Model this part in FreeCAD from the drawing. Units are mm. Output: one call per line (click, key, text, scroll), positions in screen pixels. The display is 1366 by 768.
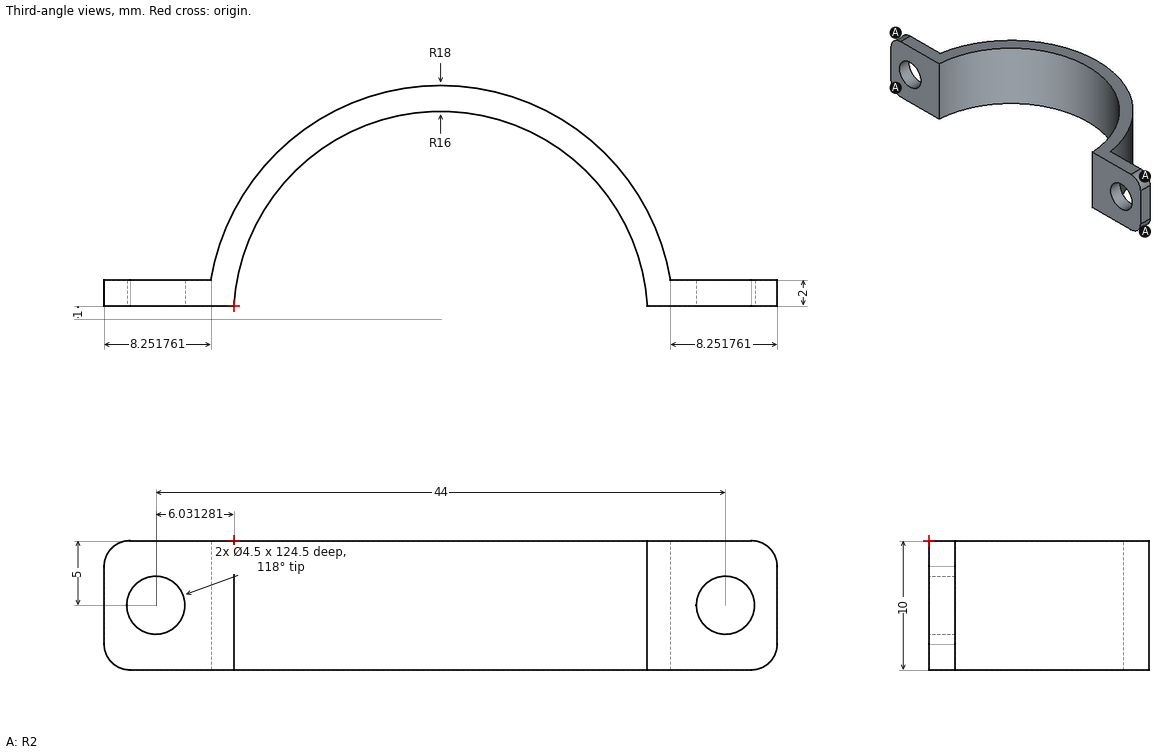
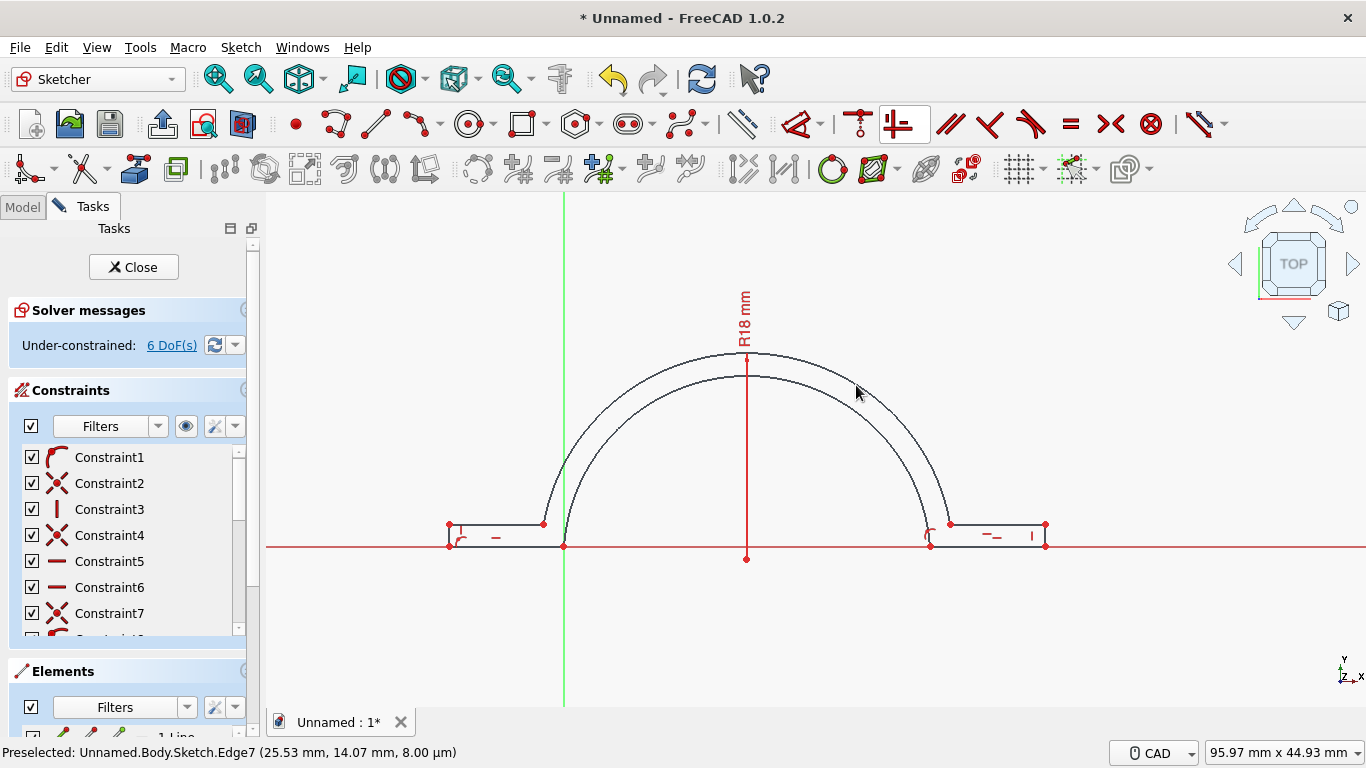
click(851, 408)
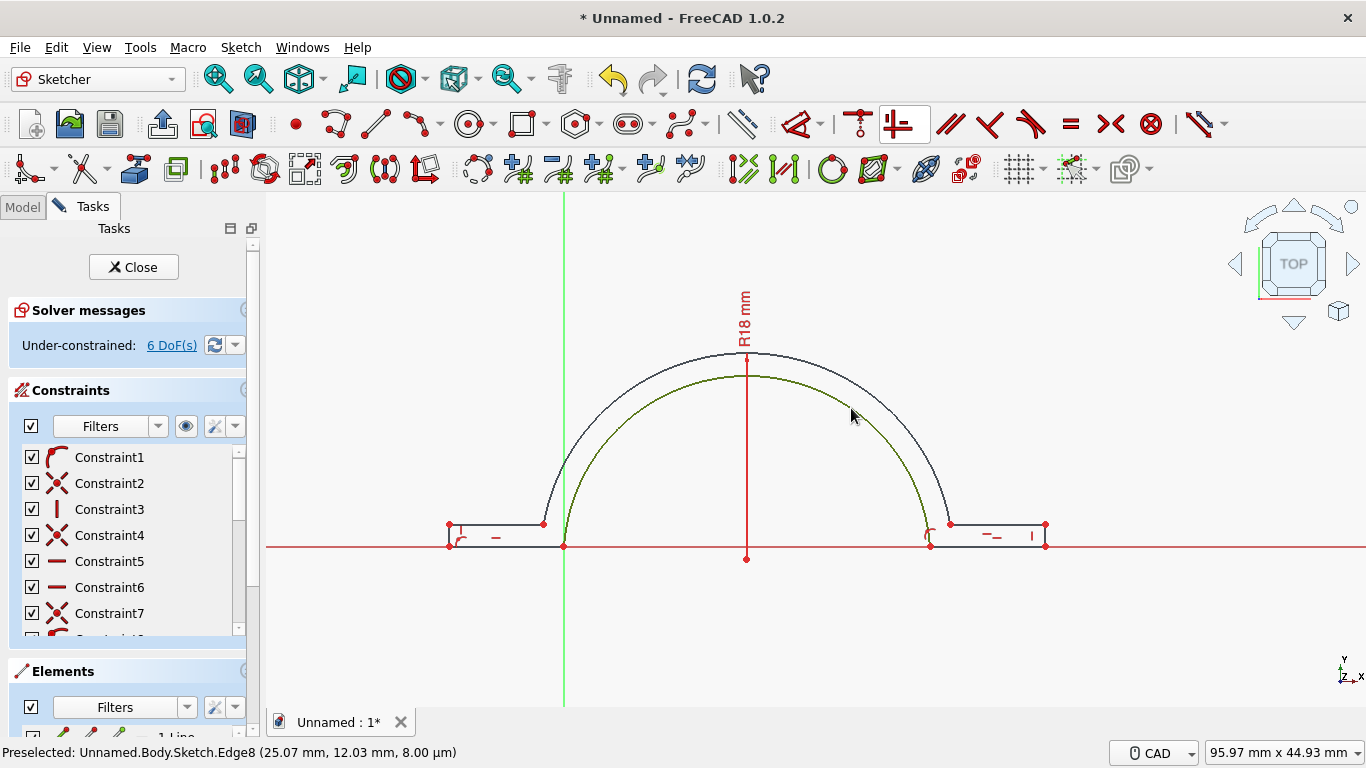
key(k)
key(r)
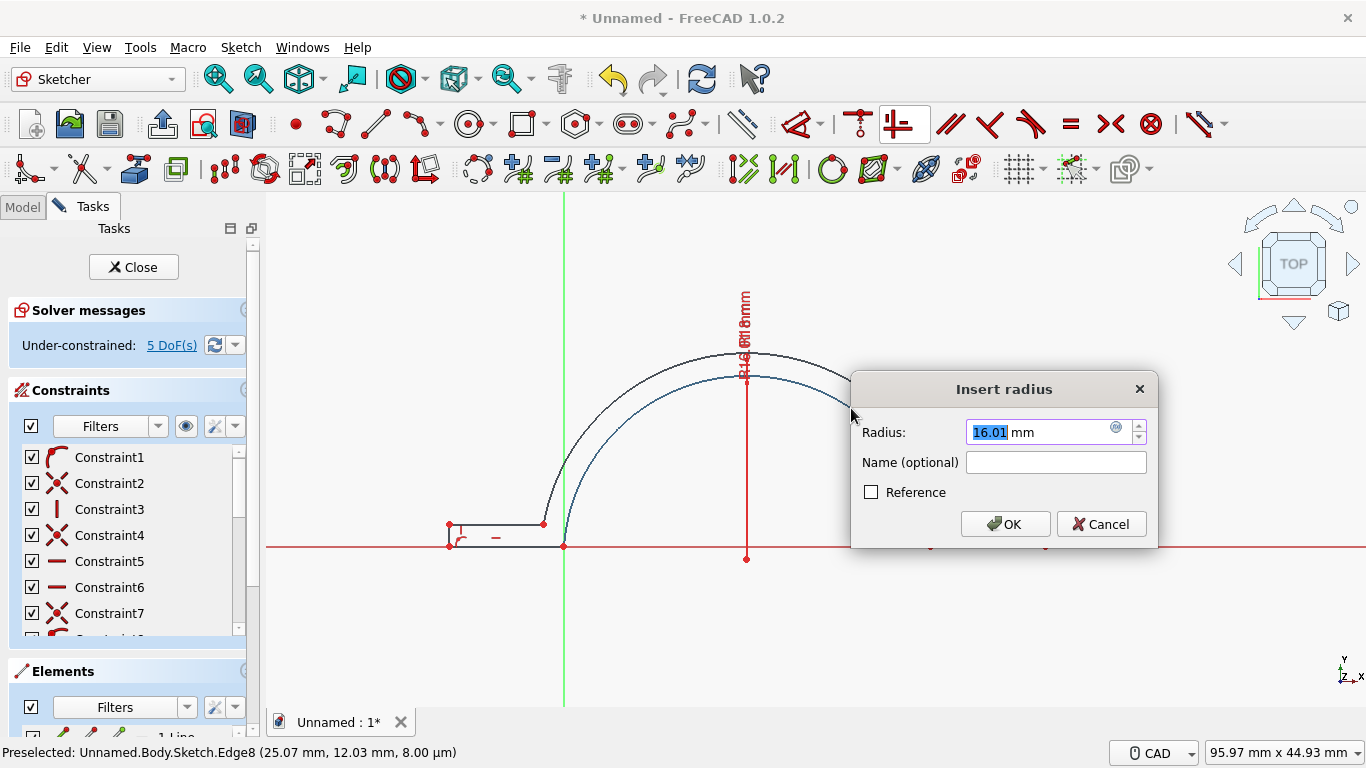
text(16)
key(Return)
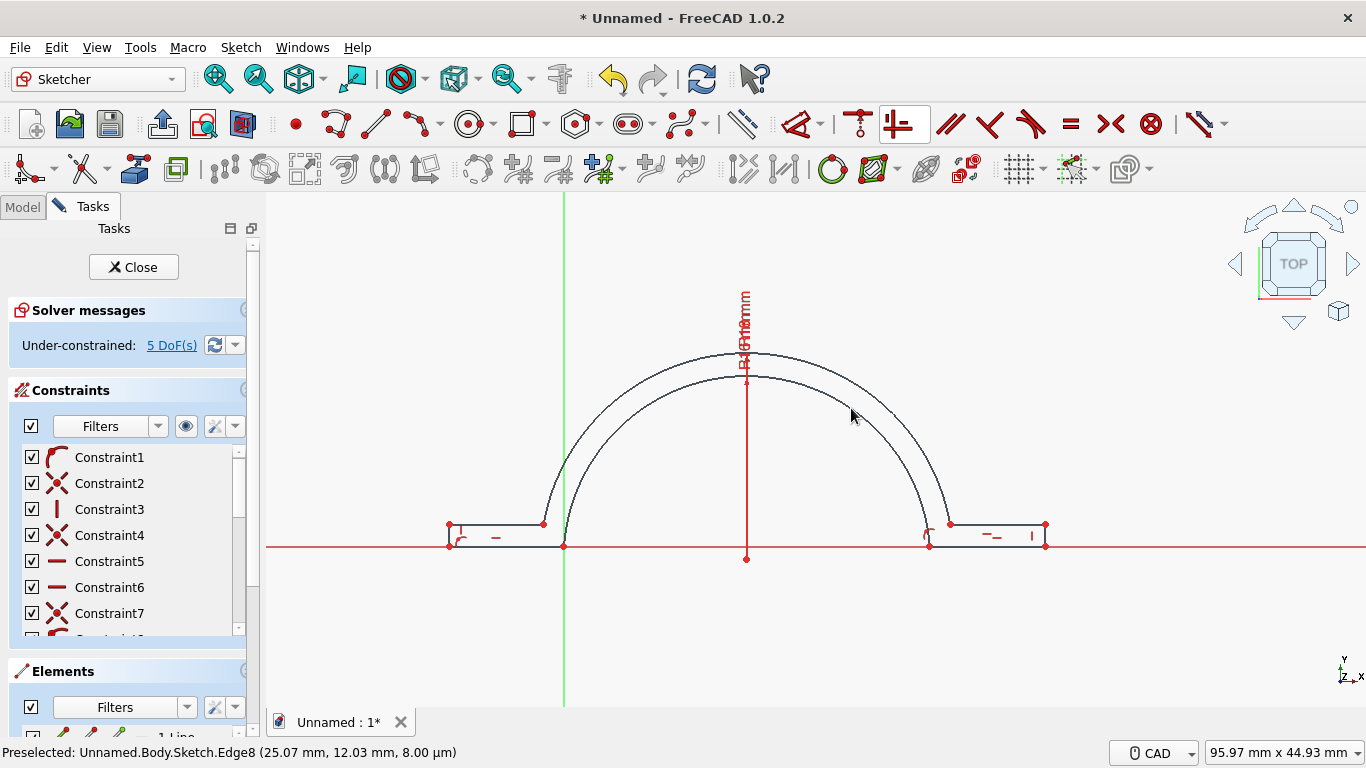
scroll(1045, 536, up, 3)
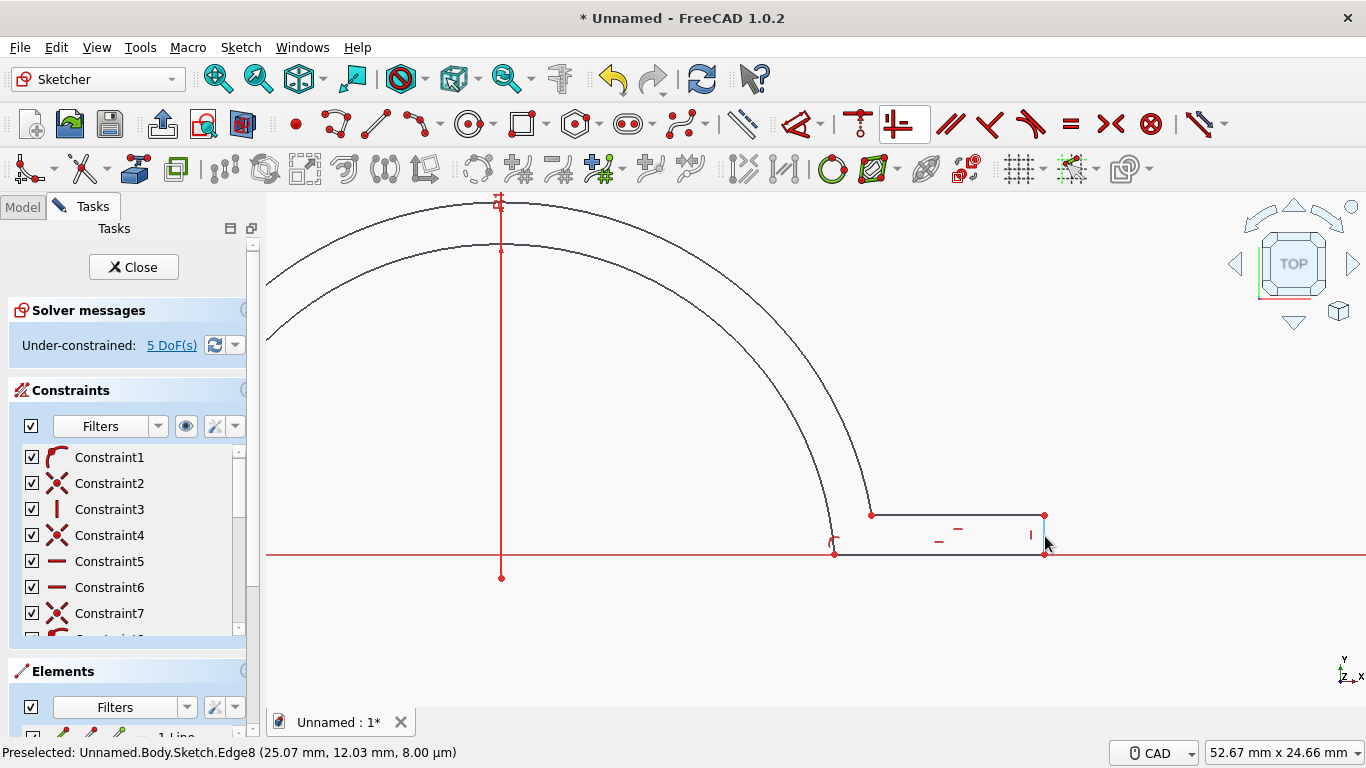
click(1044, 535)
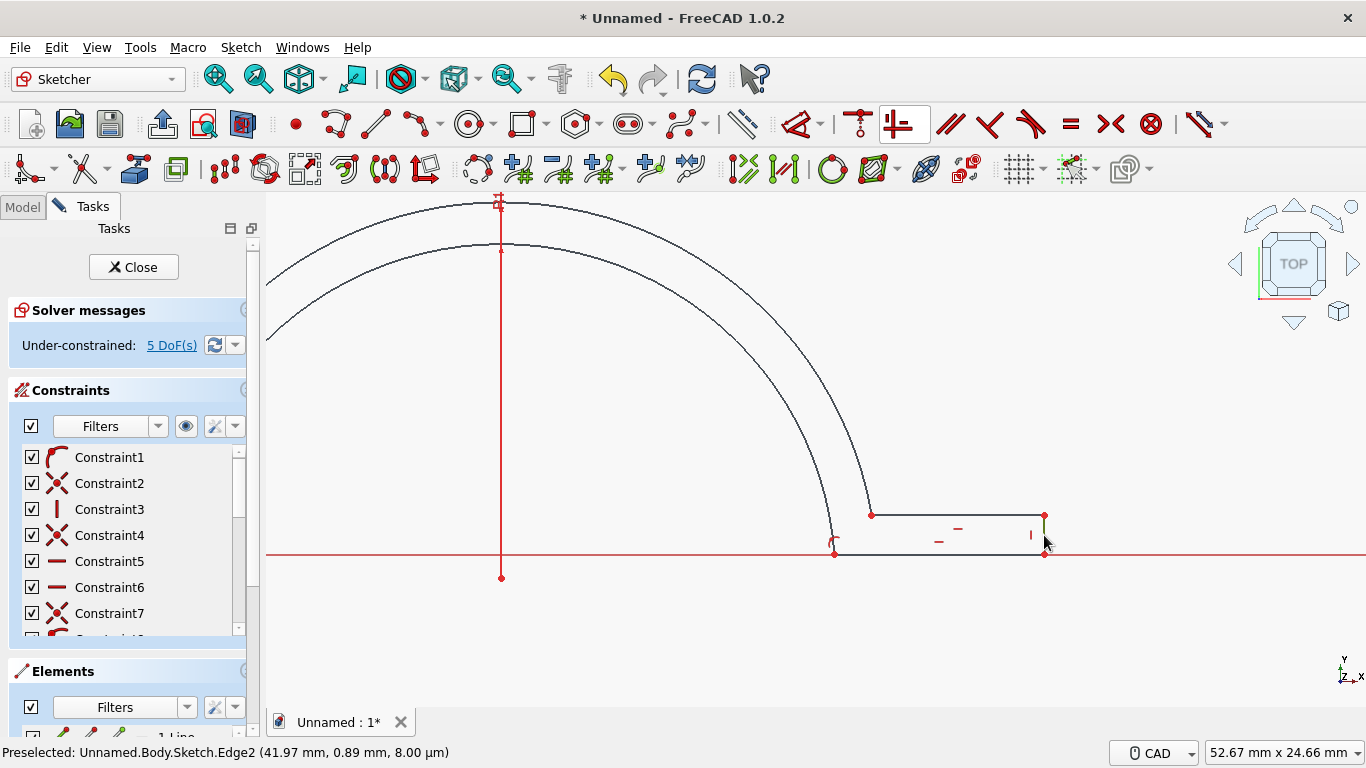
key(i)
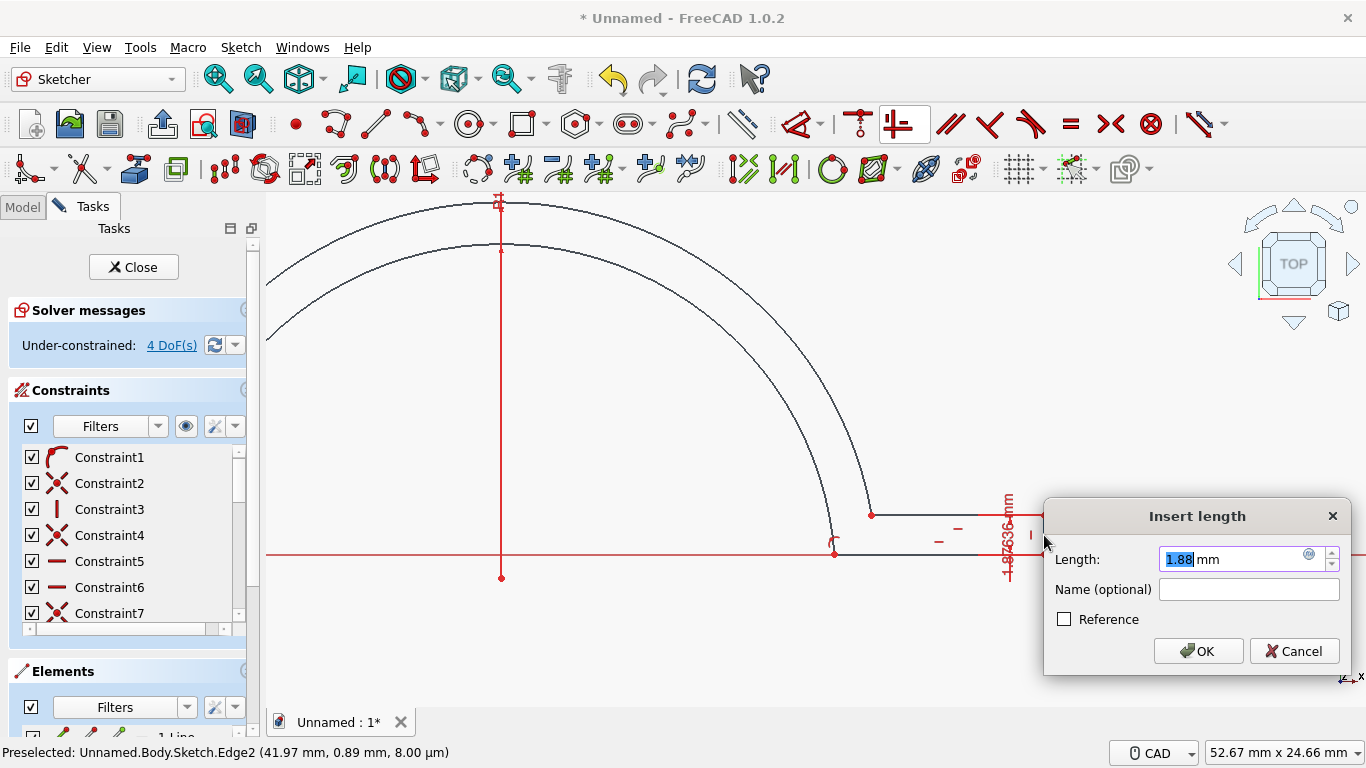
text(2)
key(Return)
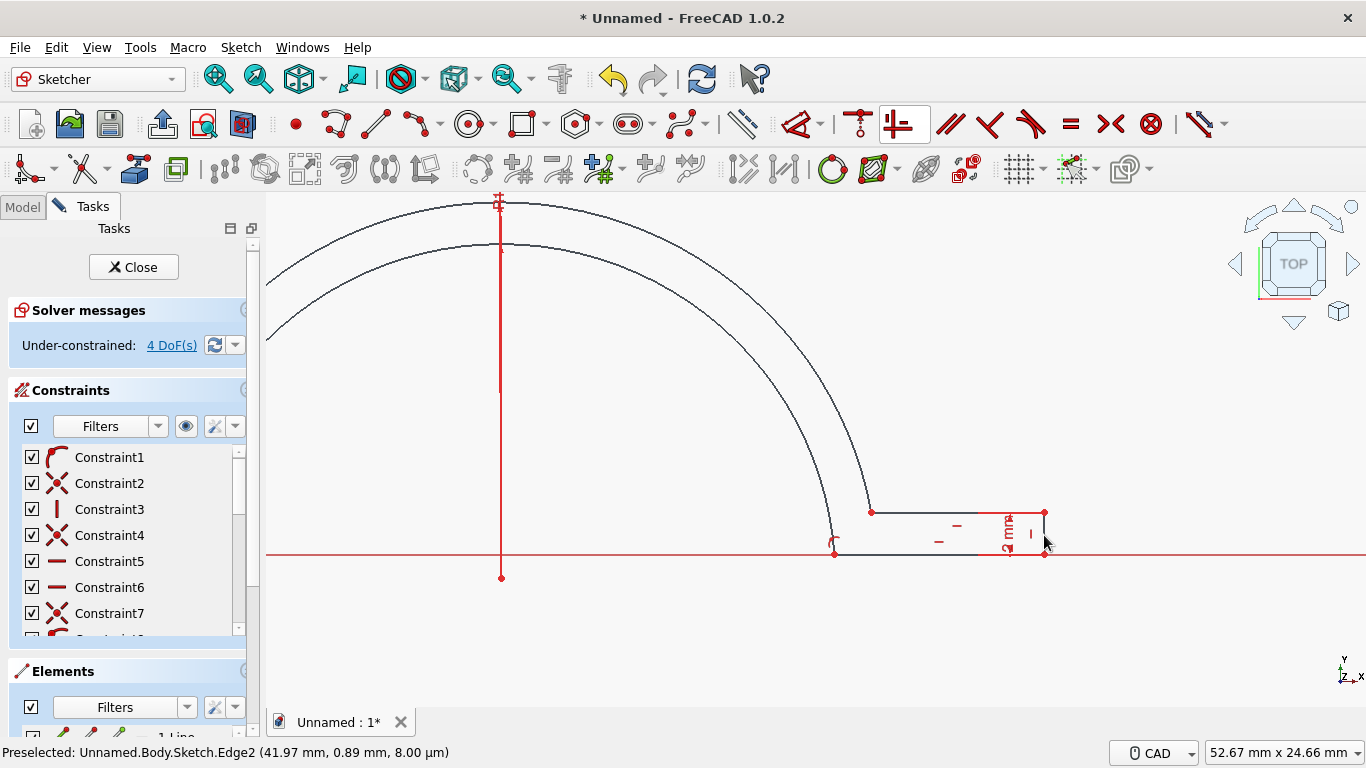
scroll(1047, 538, down, 3)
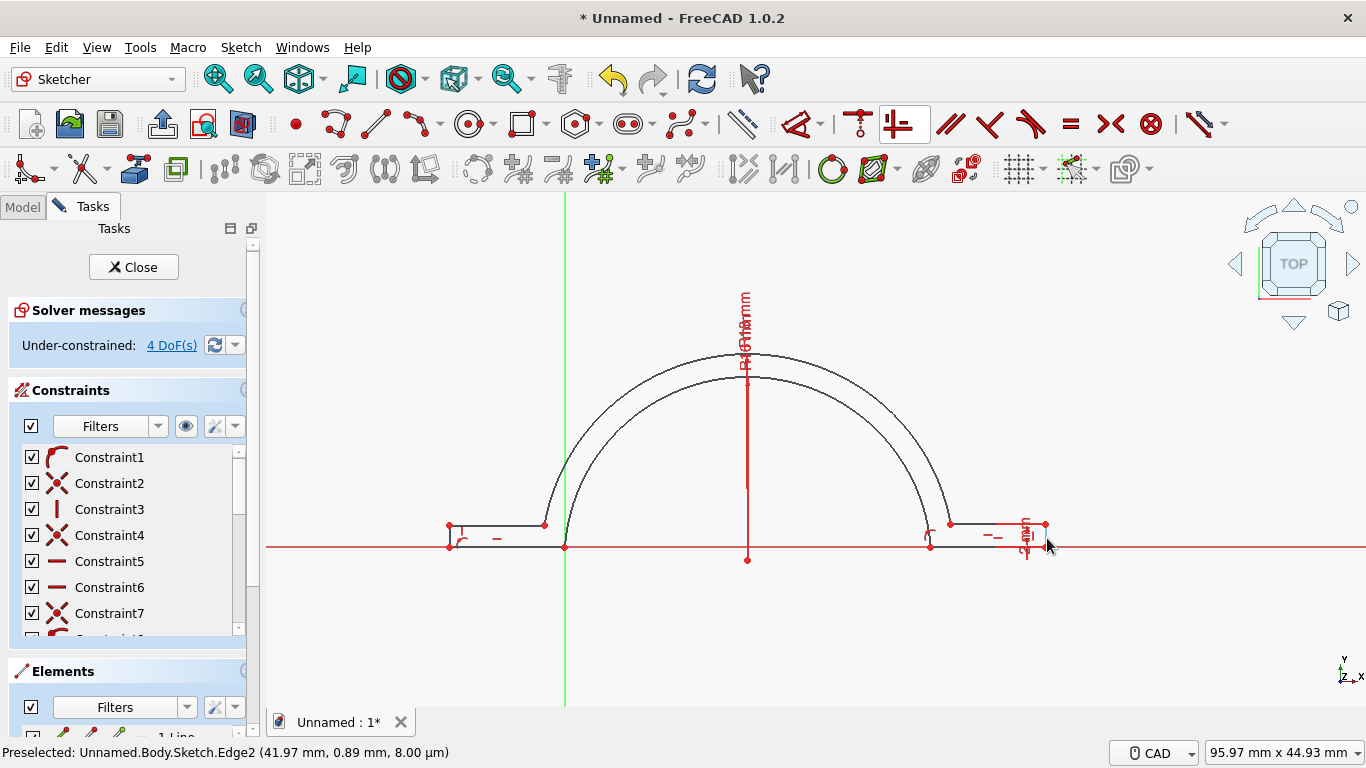
scroll(450, 532, up, 4)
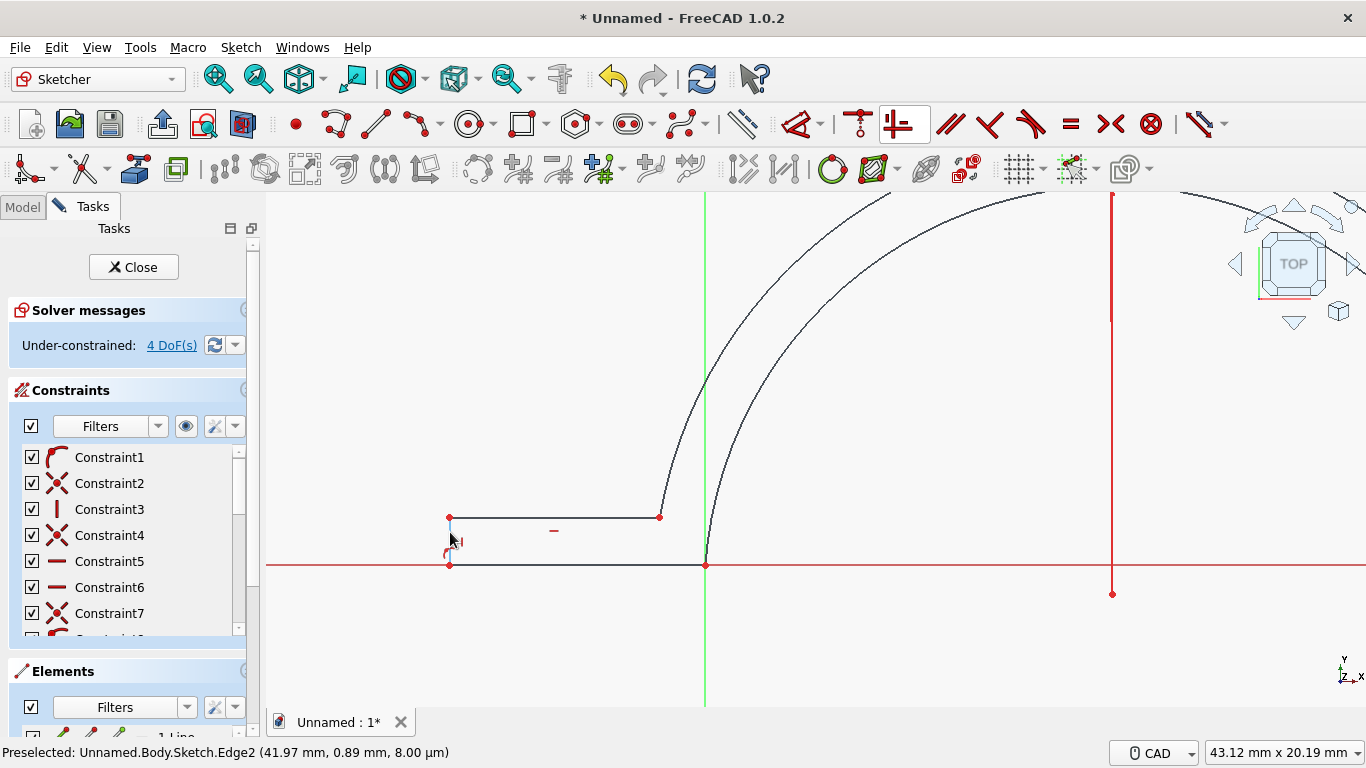
click(450, 532)